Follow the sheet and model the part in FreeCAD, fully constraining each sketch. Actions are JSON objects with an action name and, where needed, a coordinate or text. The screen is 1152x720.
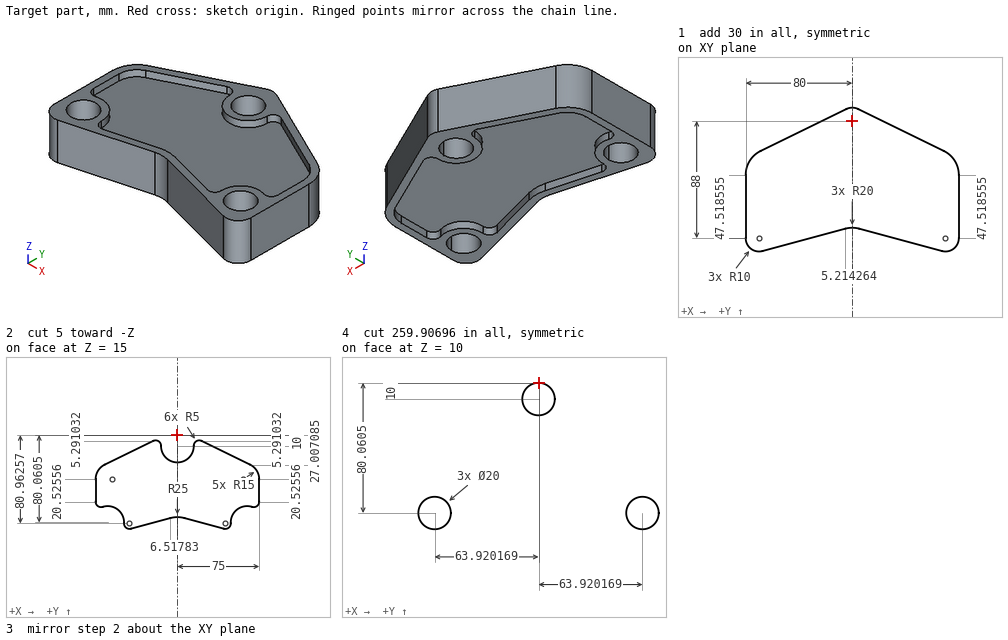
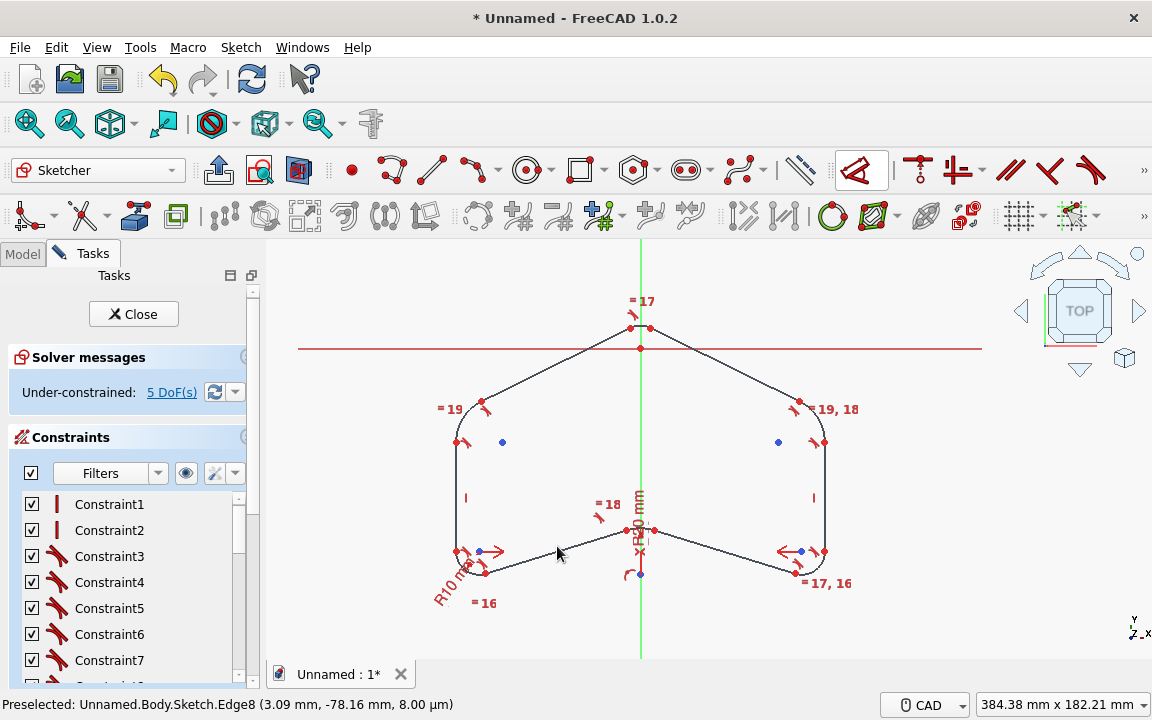
{"action": "left_click", "coordinate": [456, 443]}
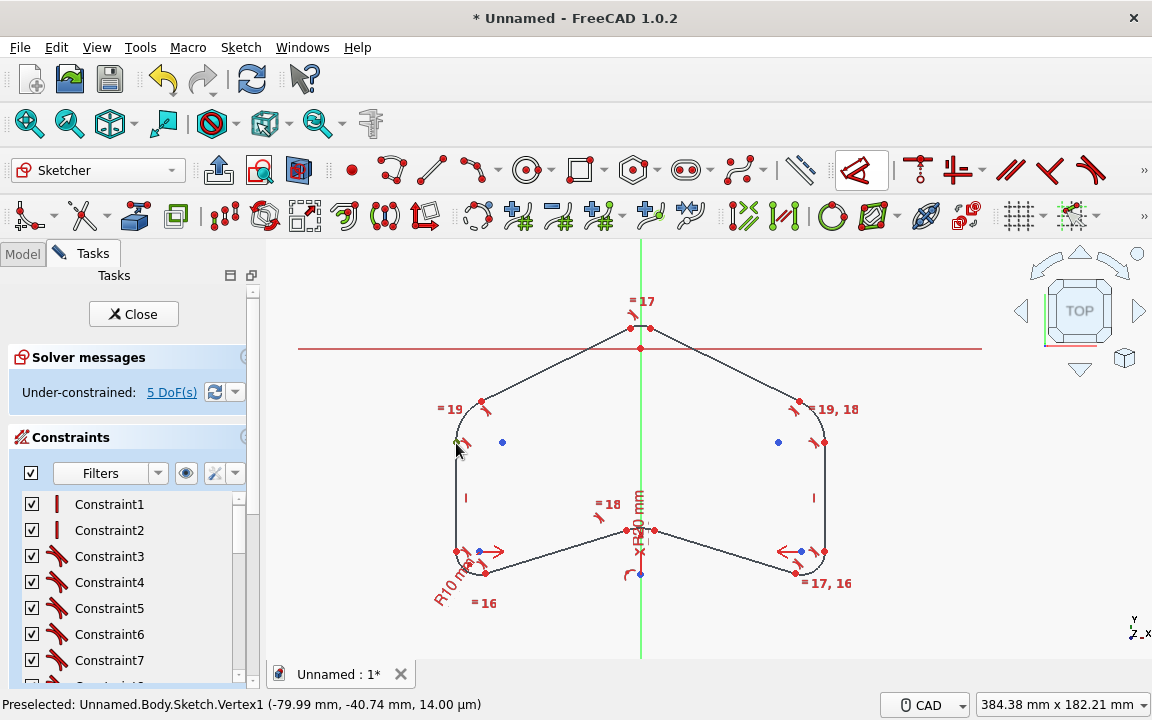
{"action": "left_click", "coordinate": [882, 170]}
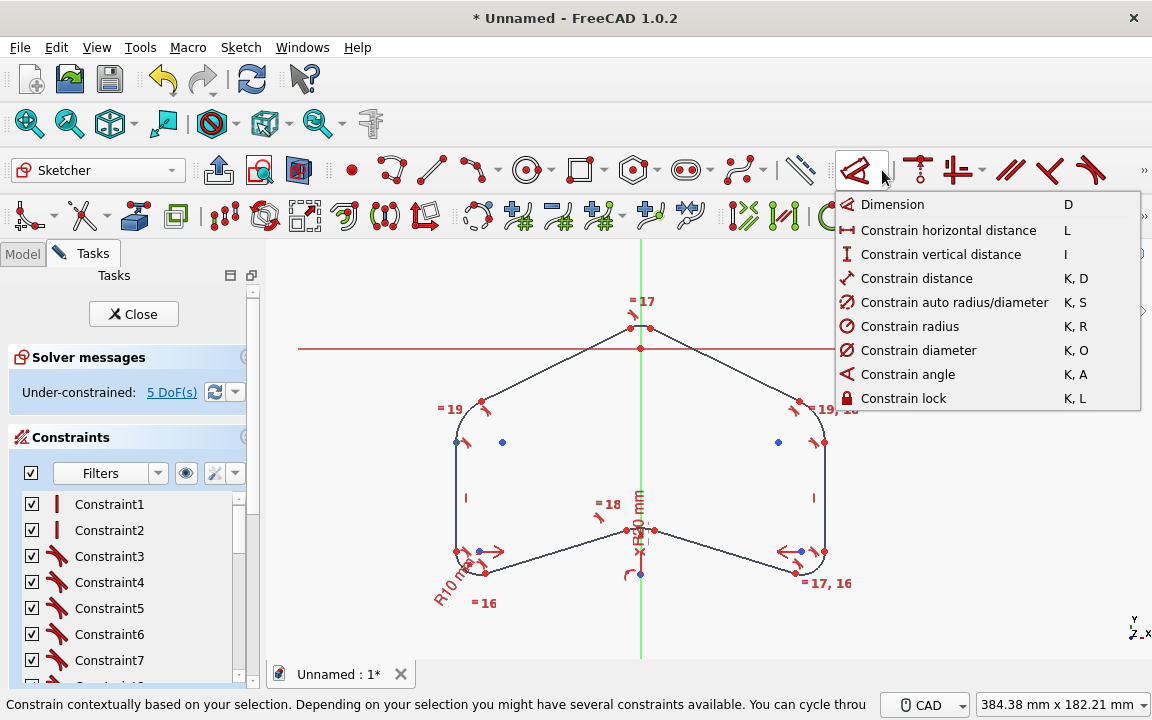
{"action": "left_click", "coordinate": [988, 230]}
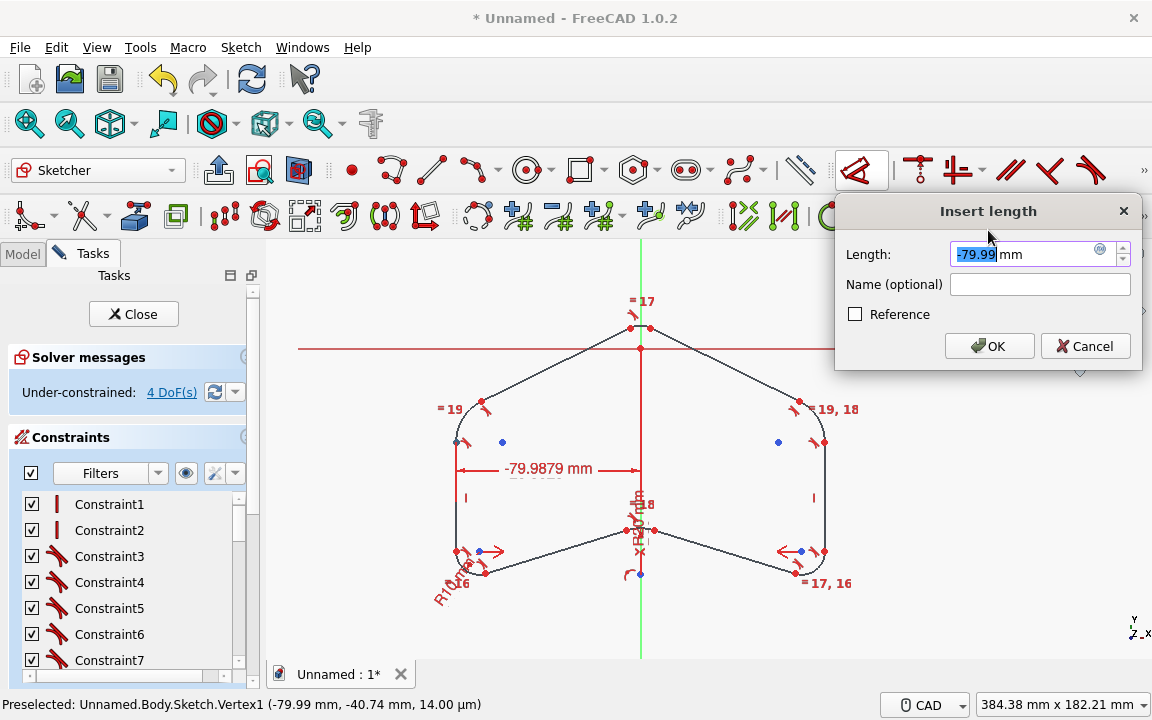
{"action": "type", "text": "-80"}
{"action": "key", "text": "Return"}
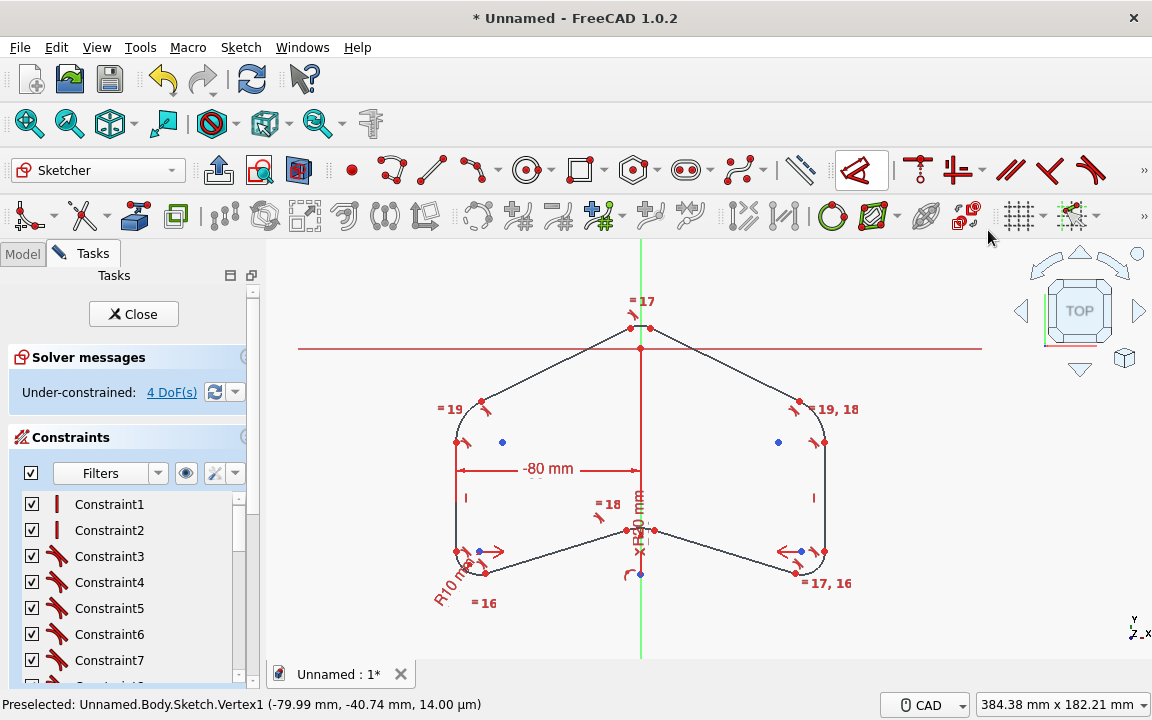
{"action": "left_click", "coordinate": [456, 552]}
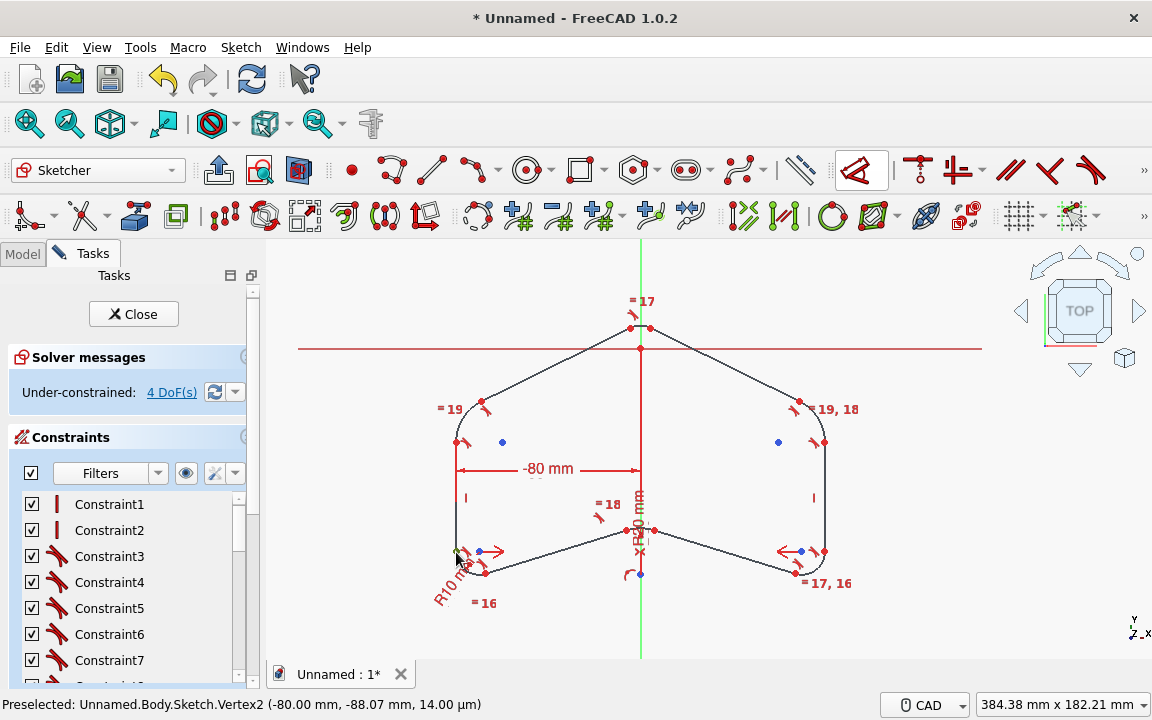
{"action": "key", "text": "i"}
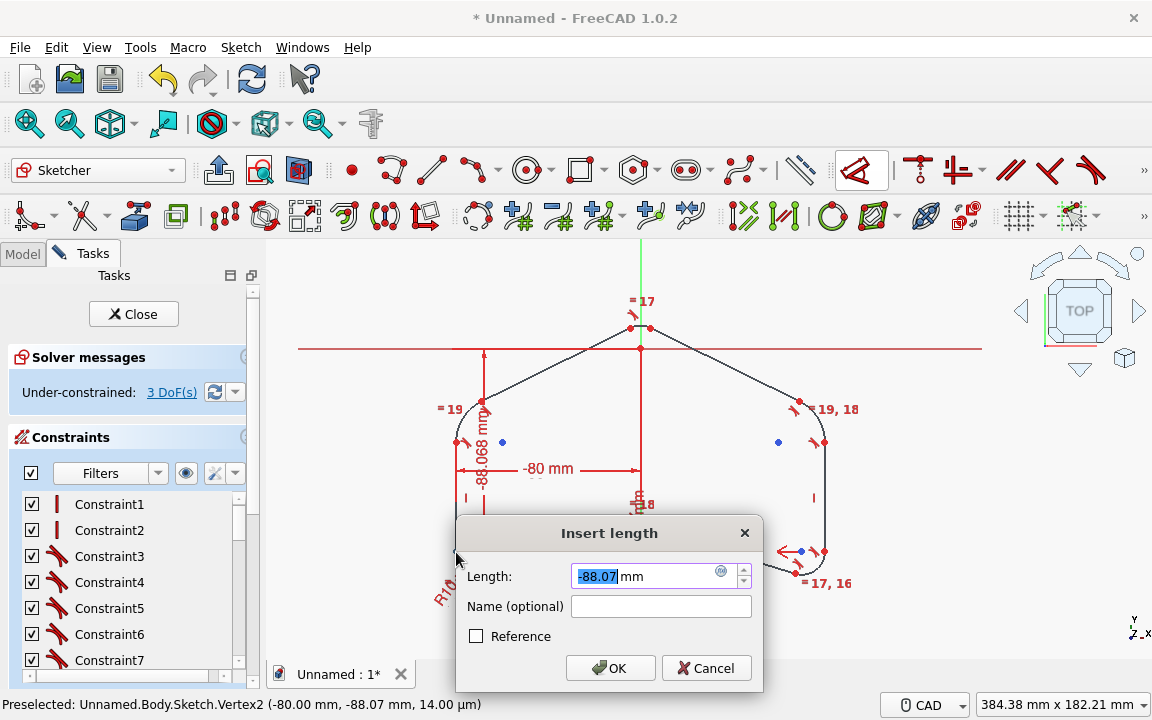
{"action": "type", "text": "-88"}
{"action": "key", "text": "Return"}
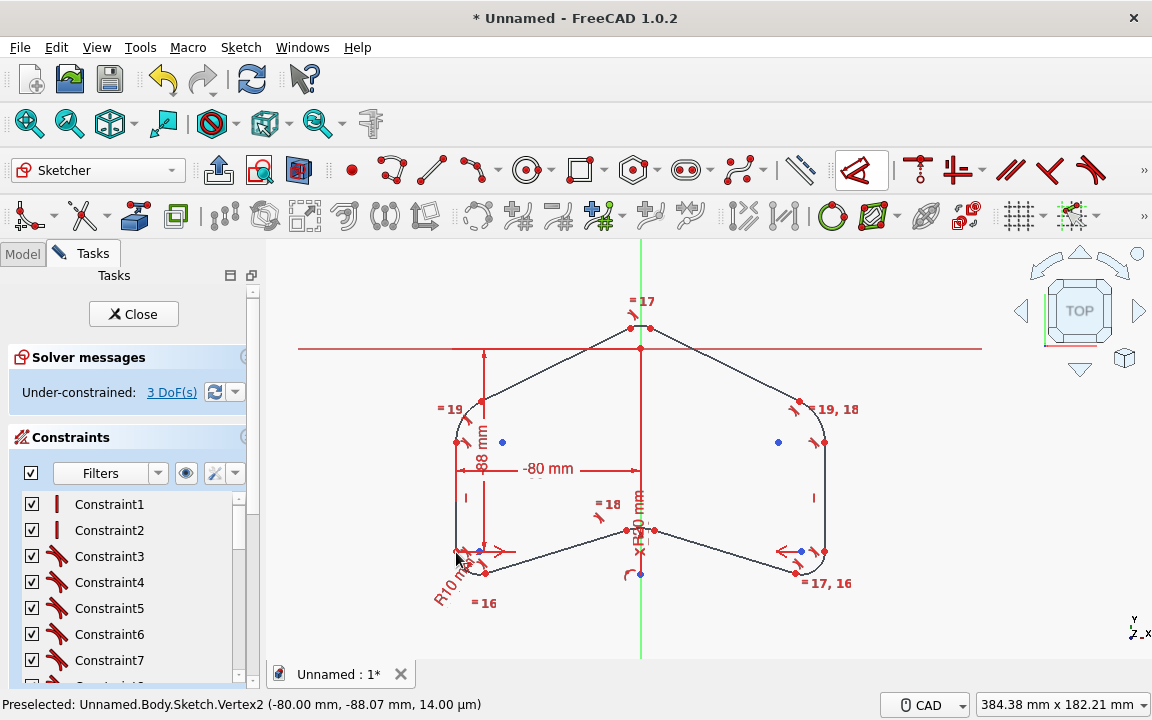
{"action": "left_click", "coordinate": [456, 475]}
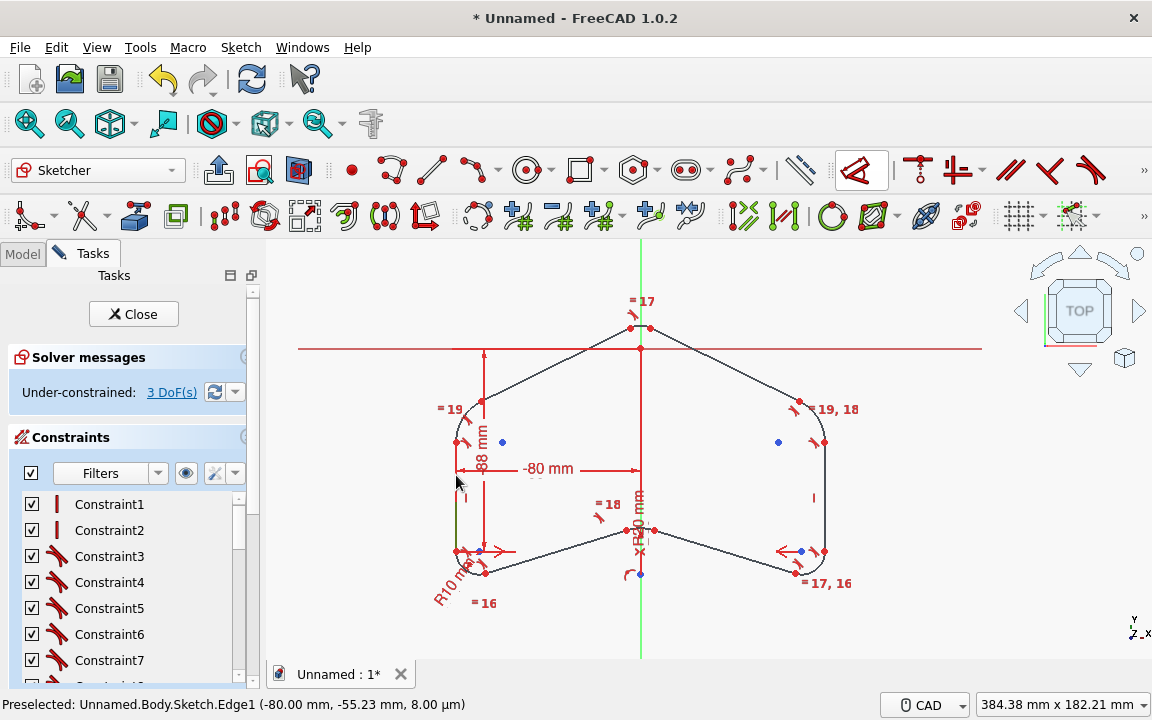
{"action": "key", "text": "i"}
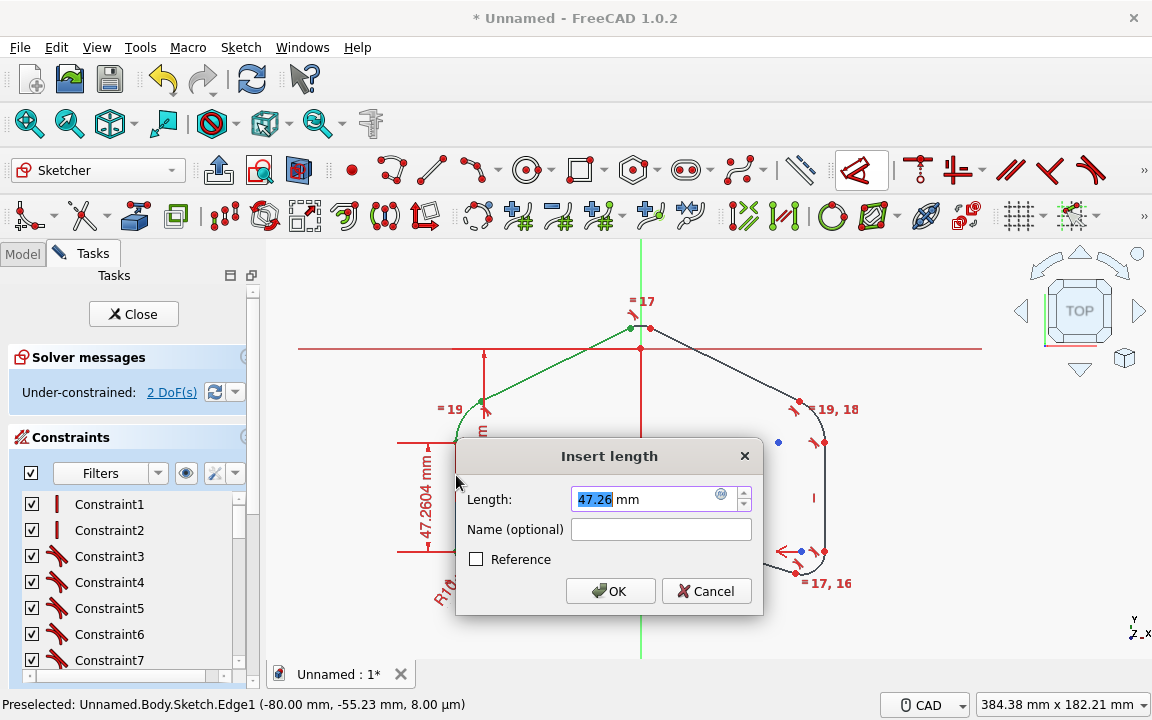
{"action": "type", "text": "47.518555"}
{"action": "key", "text": "Return"}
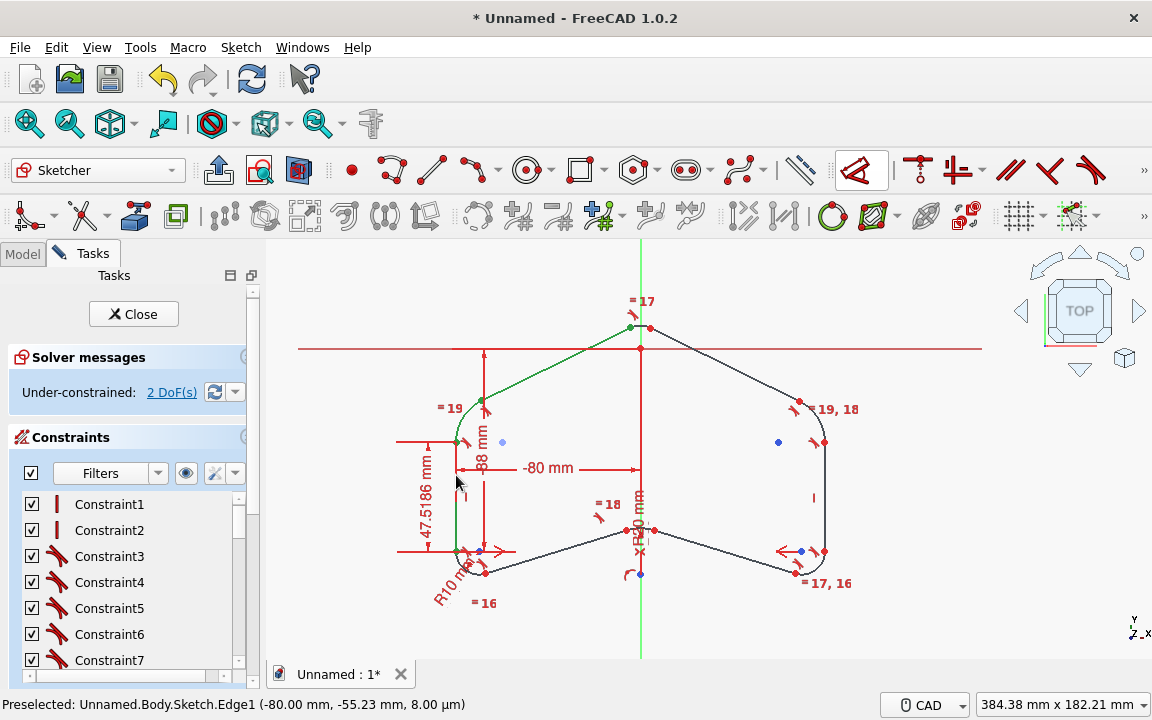
{"action": "left_click", "coordinate": [825, 519]}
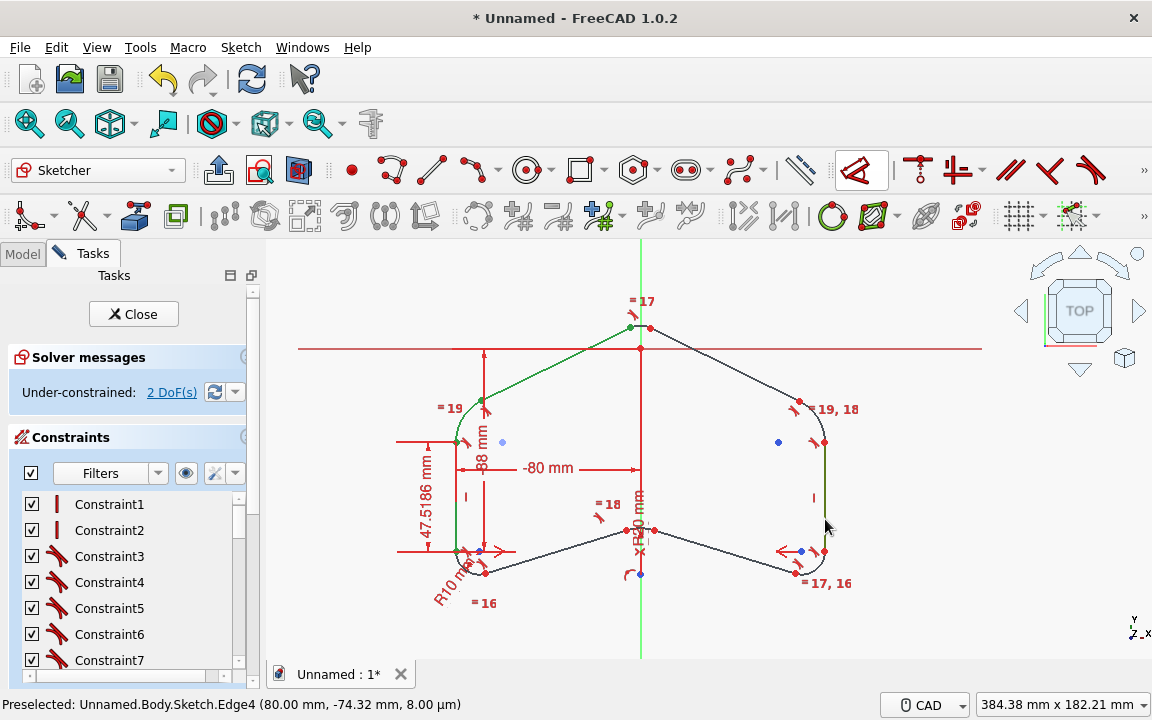
{"action": "key", "text": "i"}